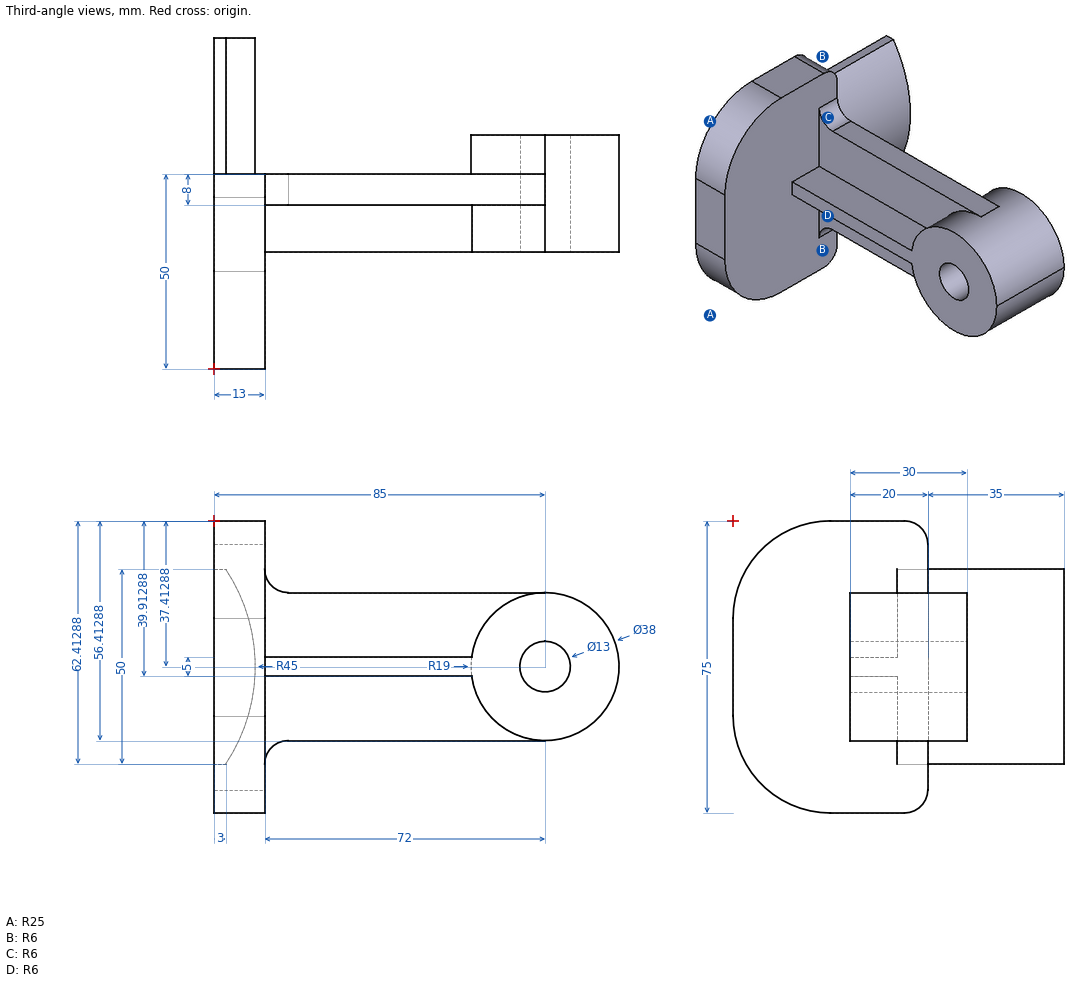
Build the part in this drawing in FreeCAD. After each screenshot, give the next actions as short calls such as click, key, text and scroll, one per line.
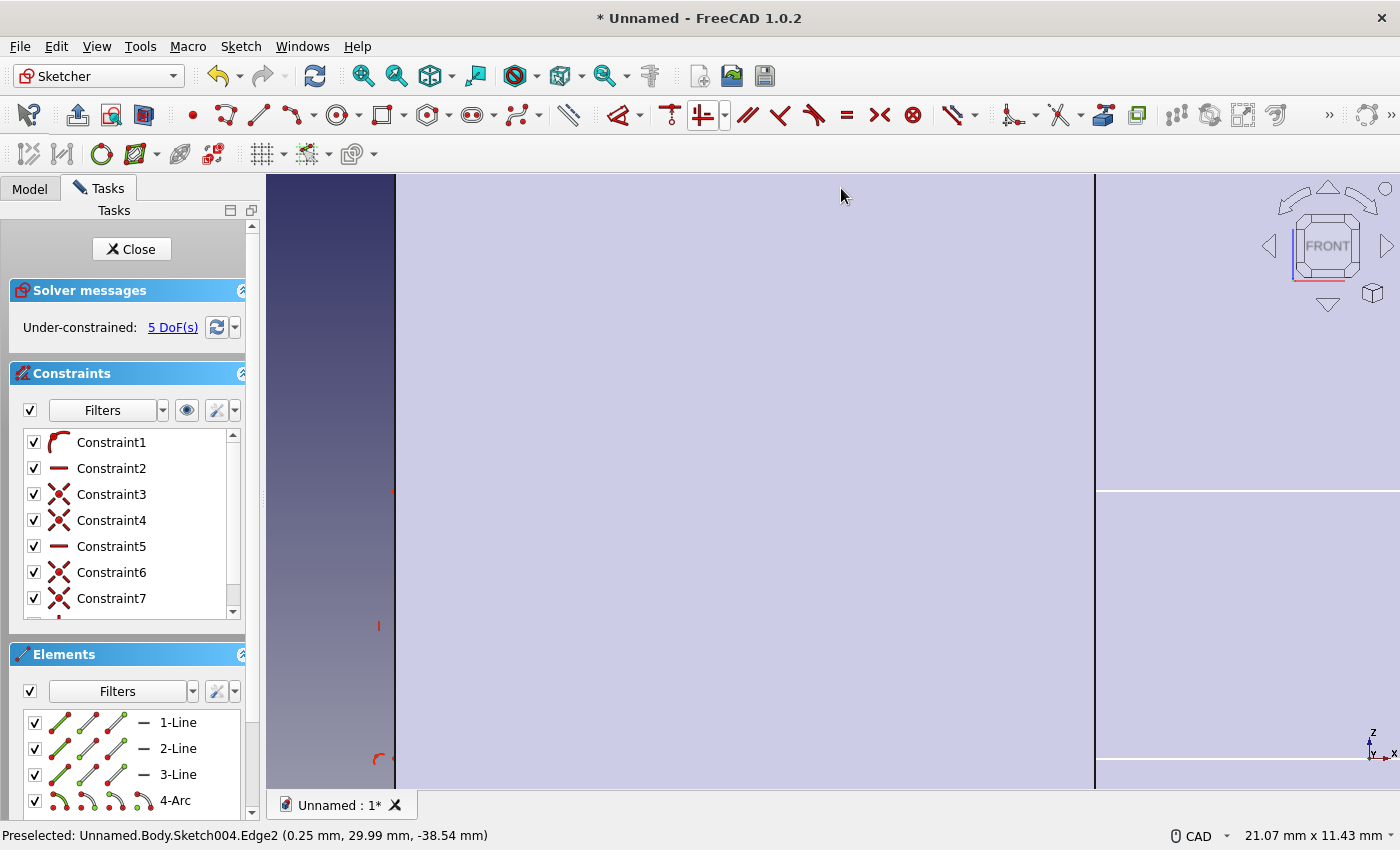
click(618, 116)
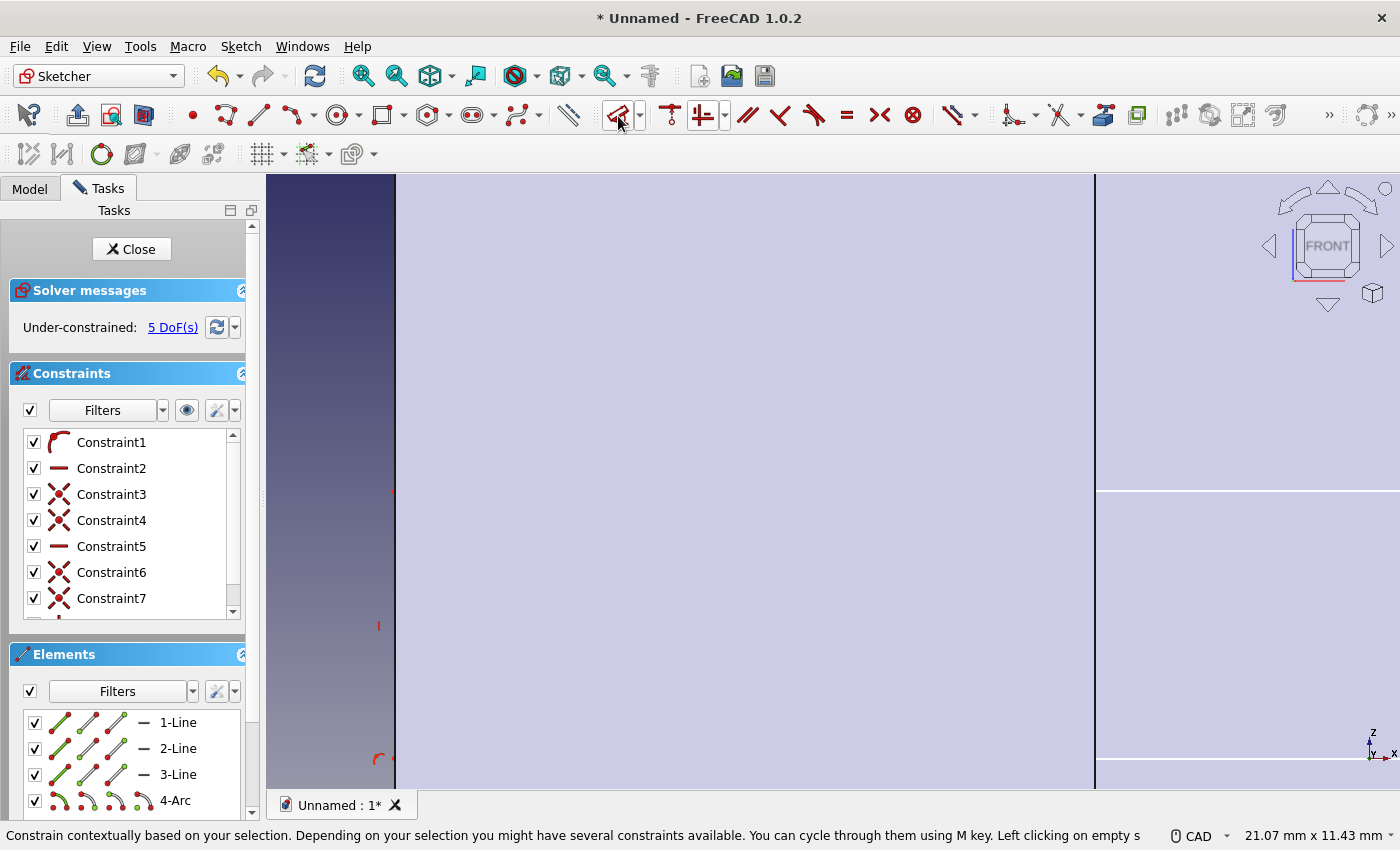
scroll(407, 684, down, 8)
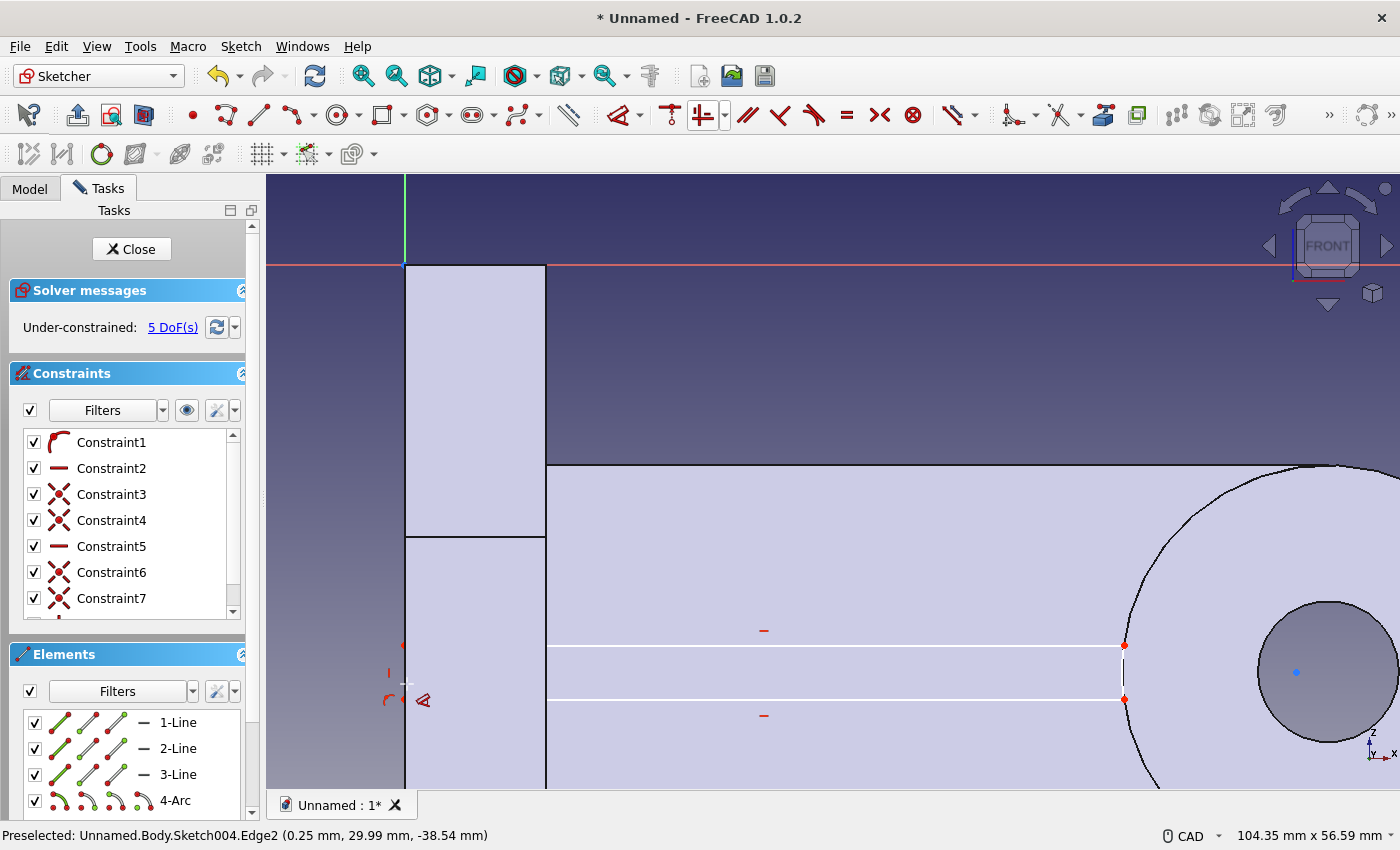
click(1122, 662)
click(1090, 660)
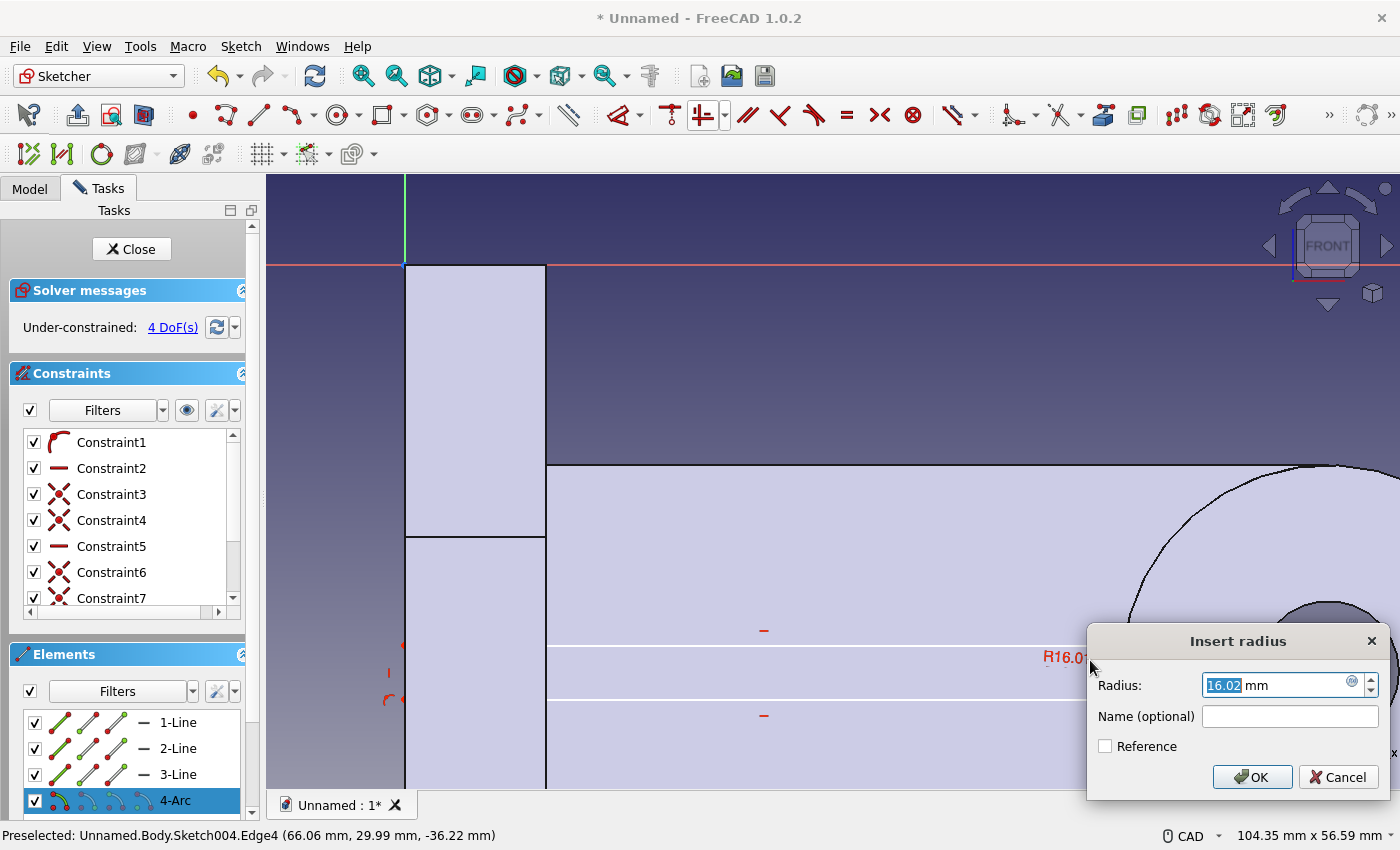
text(19)
key(Return)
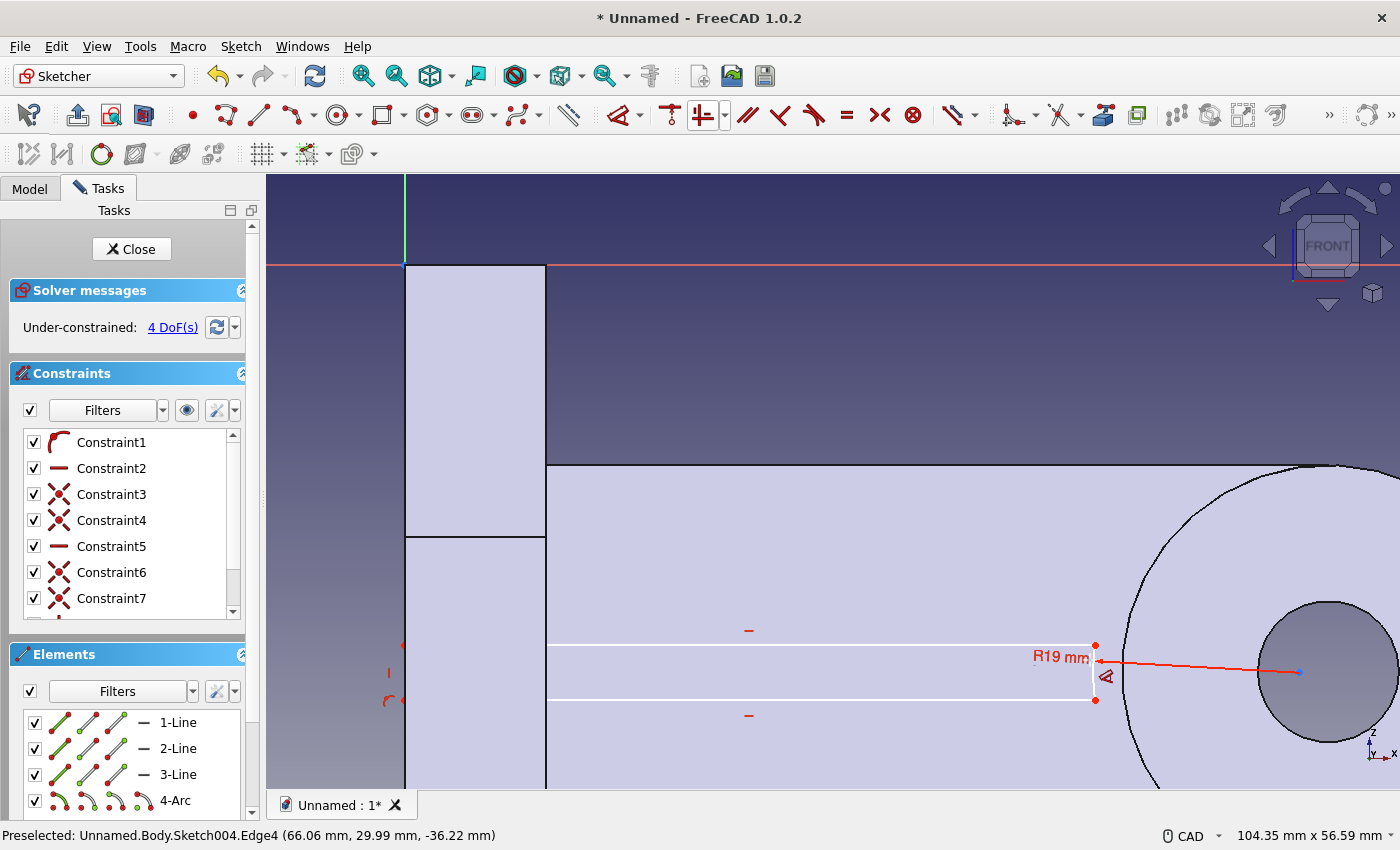
click(405, 684)
click(371, 673)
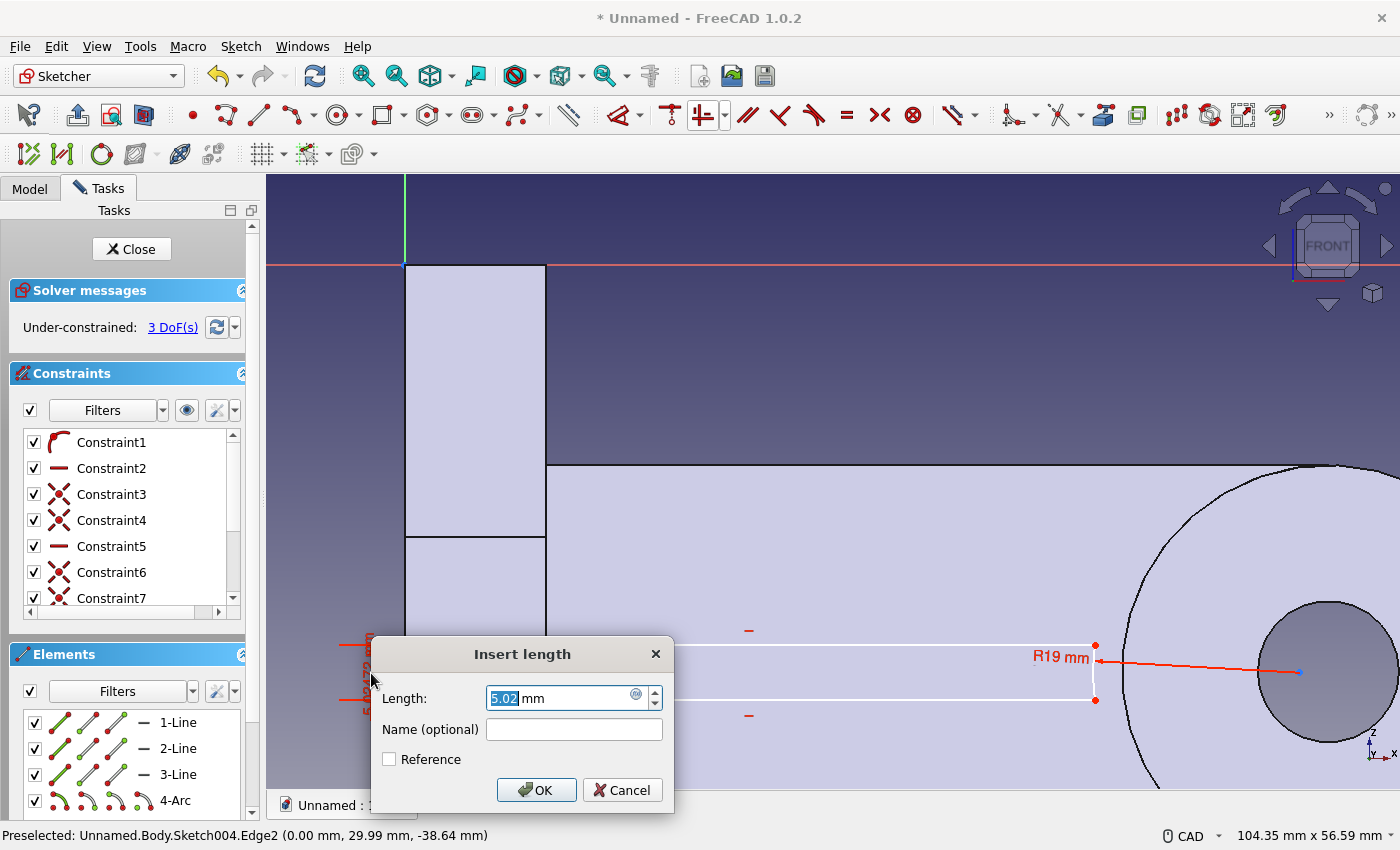
text(5)
key(Return)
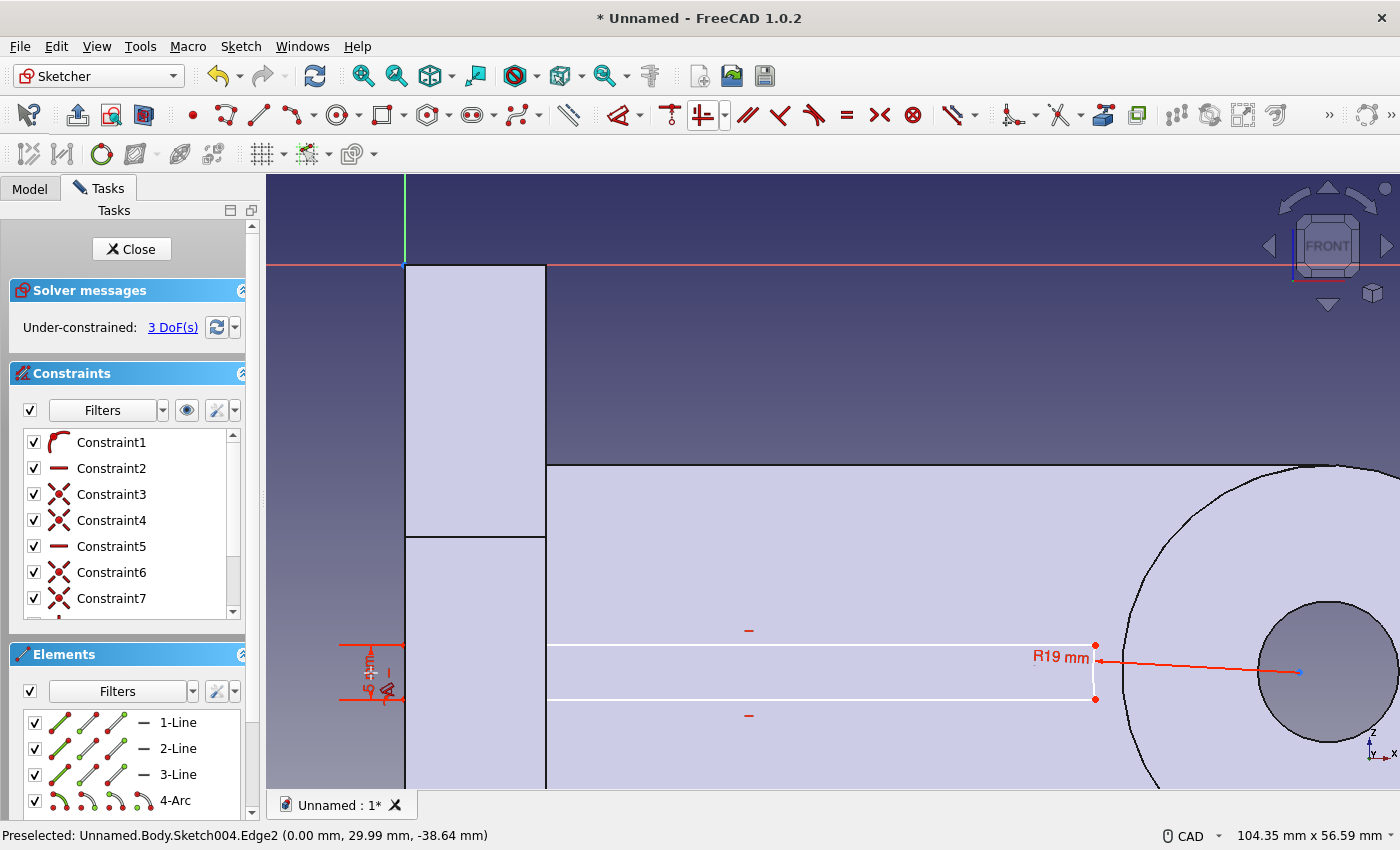
scroll(368, 479, down, 1)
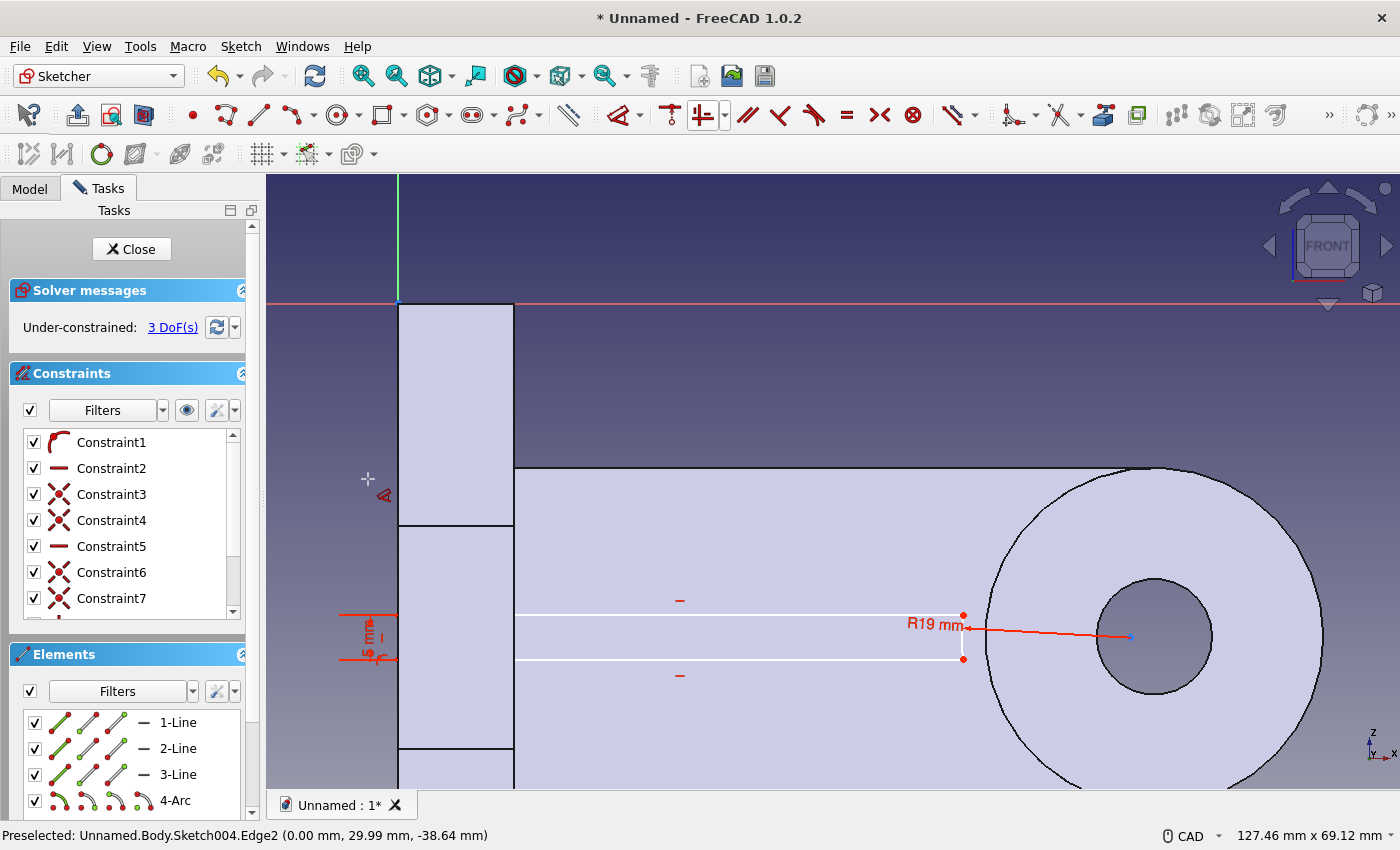
click(1131, 638)
click(764, 270)